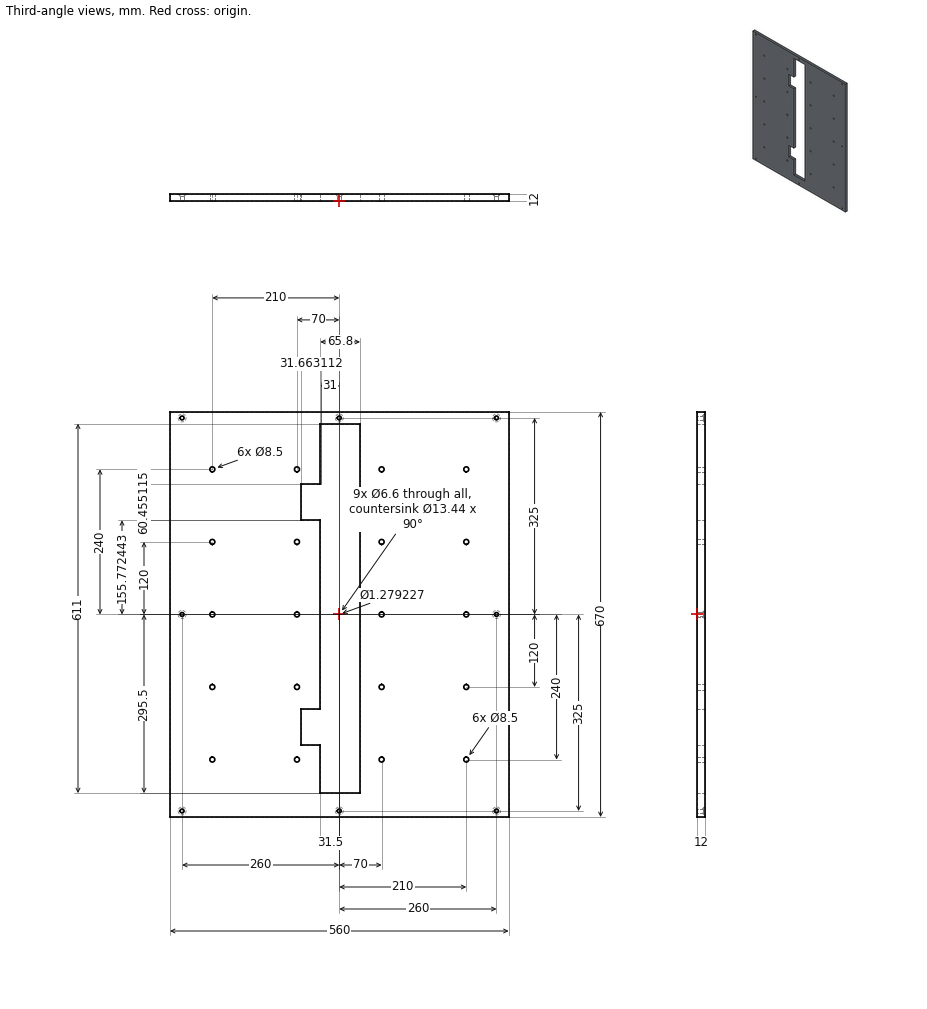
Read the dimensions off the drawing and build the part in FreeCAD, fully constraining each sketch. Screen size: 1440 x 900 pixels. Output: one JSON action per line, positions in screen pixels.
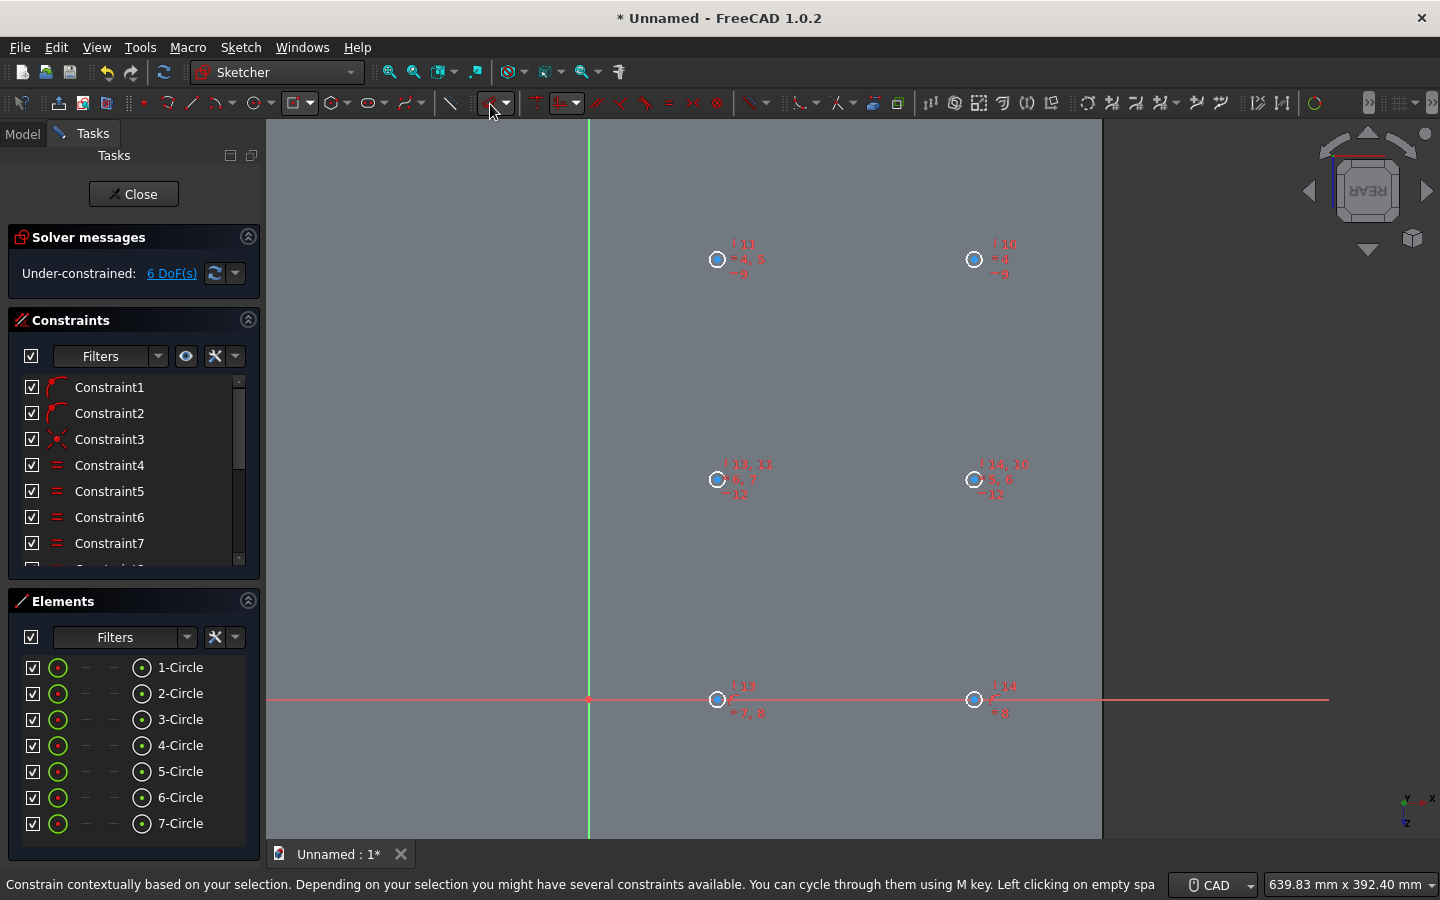
{"action": "scroll", "coordinate": [974, 267], "scroll_direction": "up", "scroll_amount": 5}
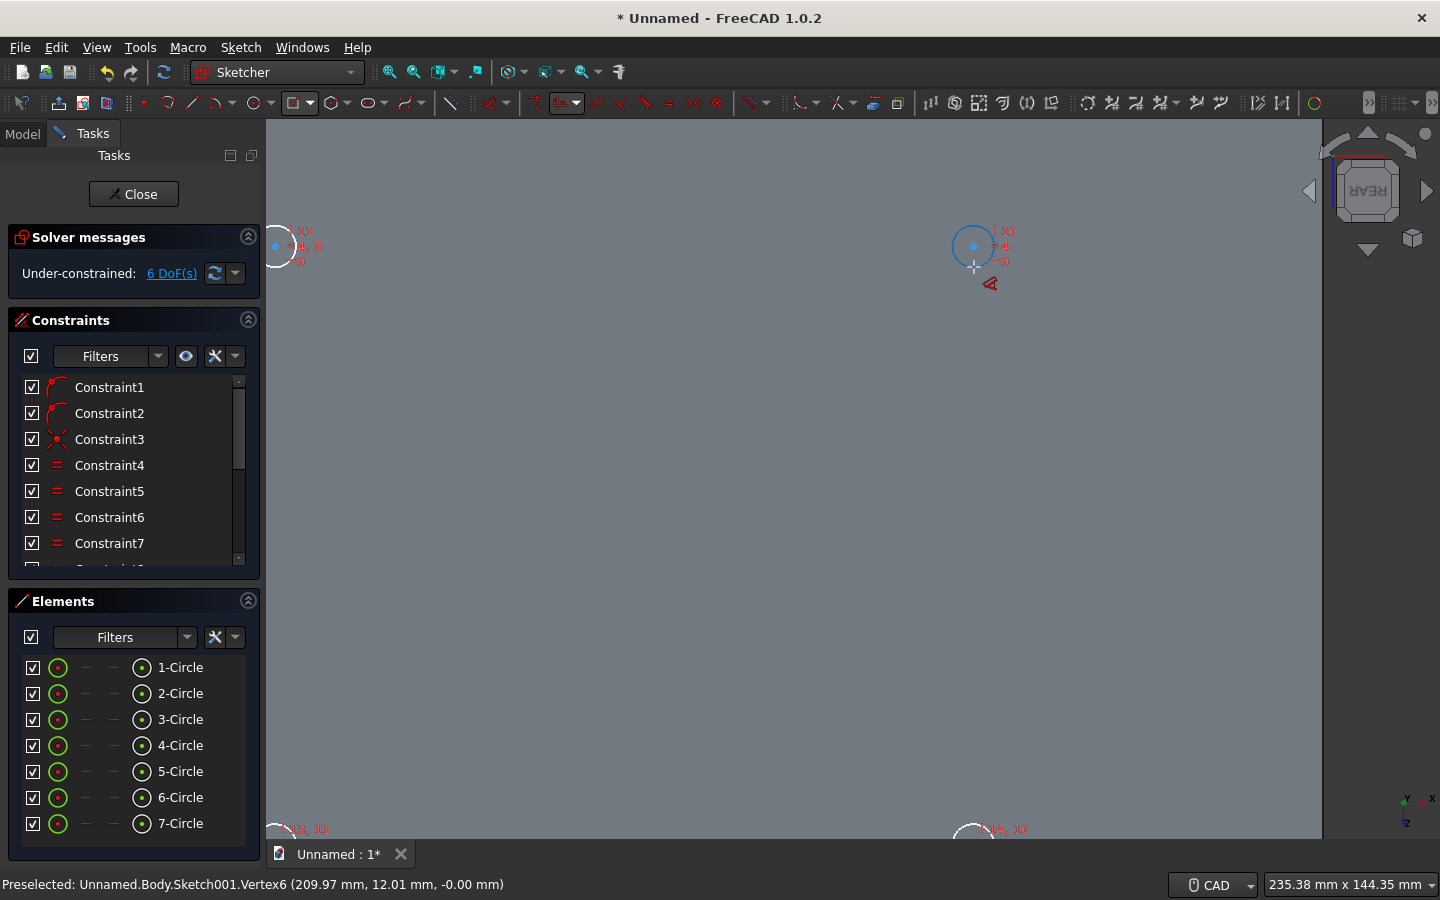
{"action": "left_click", "coordinate": [973, 267]}
{"action": "left_click", "coordinate": [973, 299]}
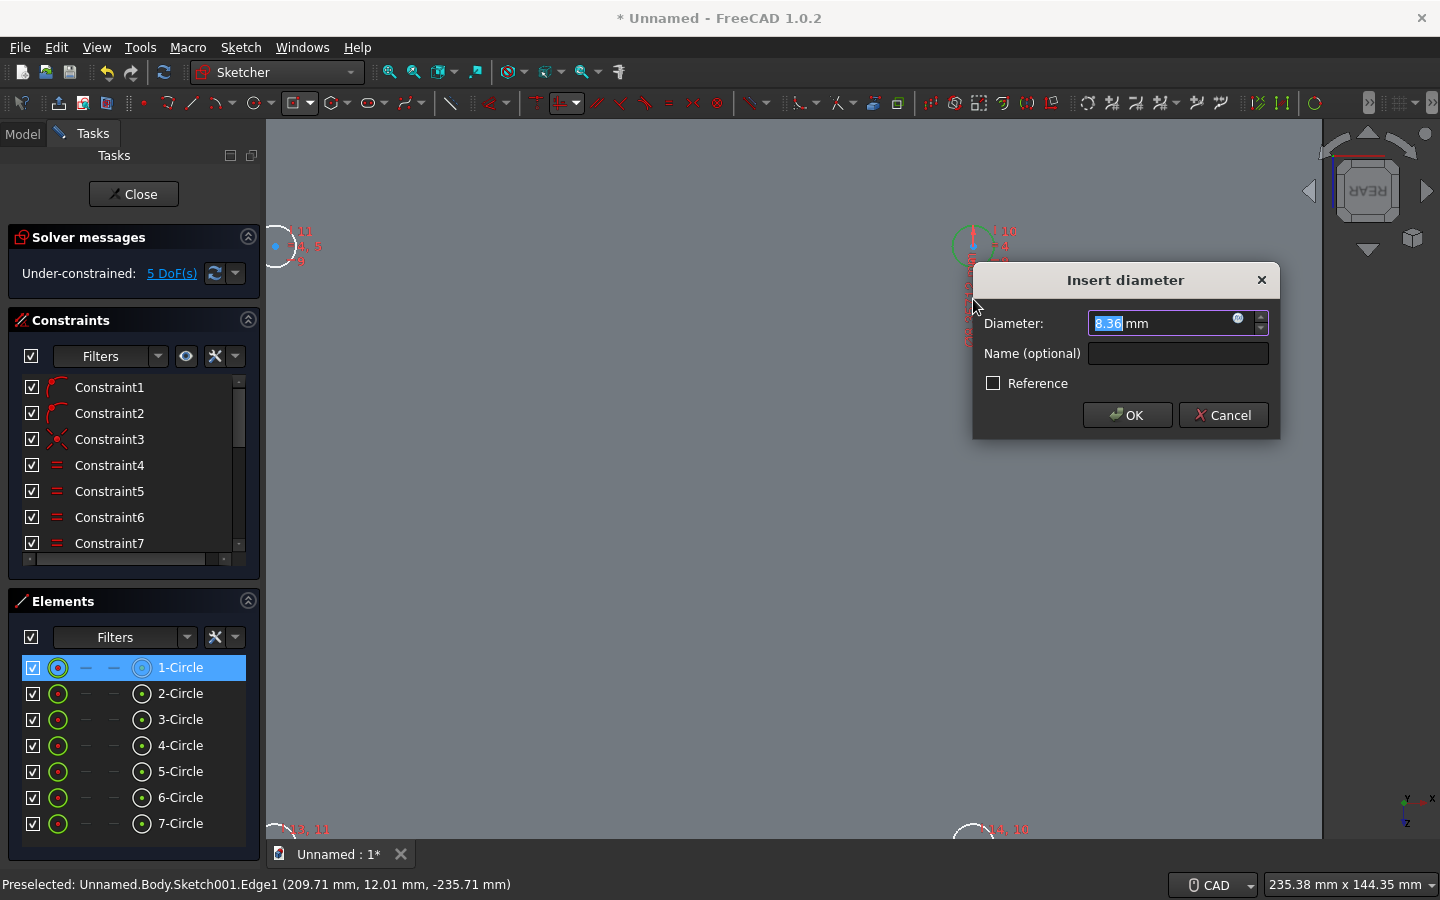
{"action": "type", "text": "8.5"}
{"action": "key", "text": "Return"}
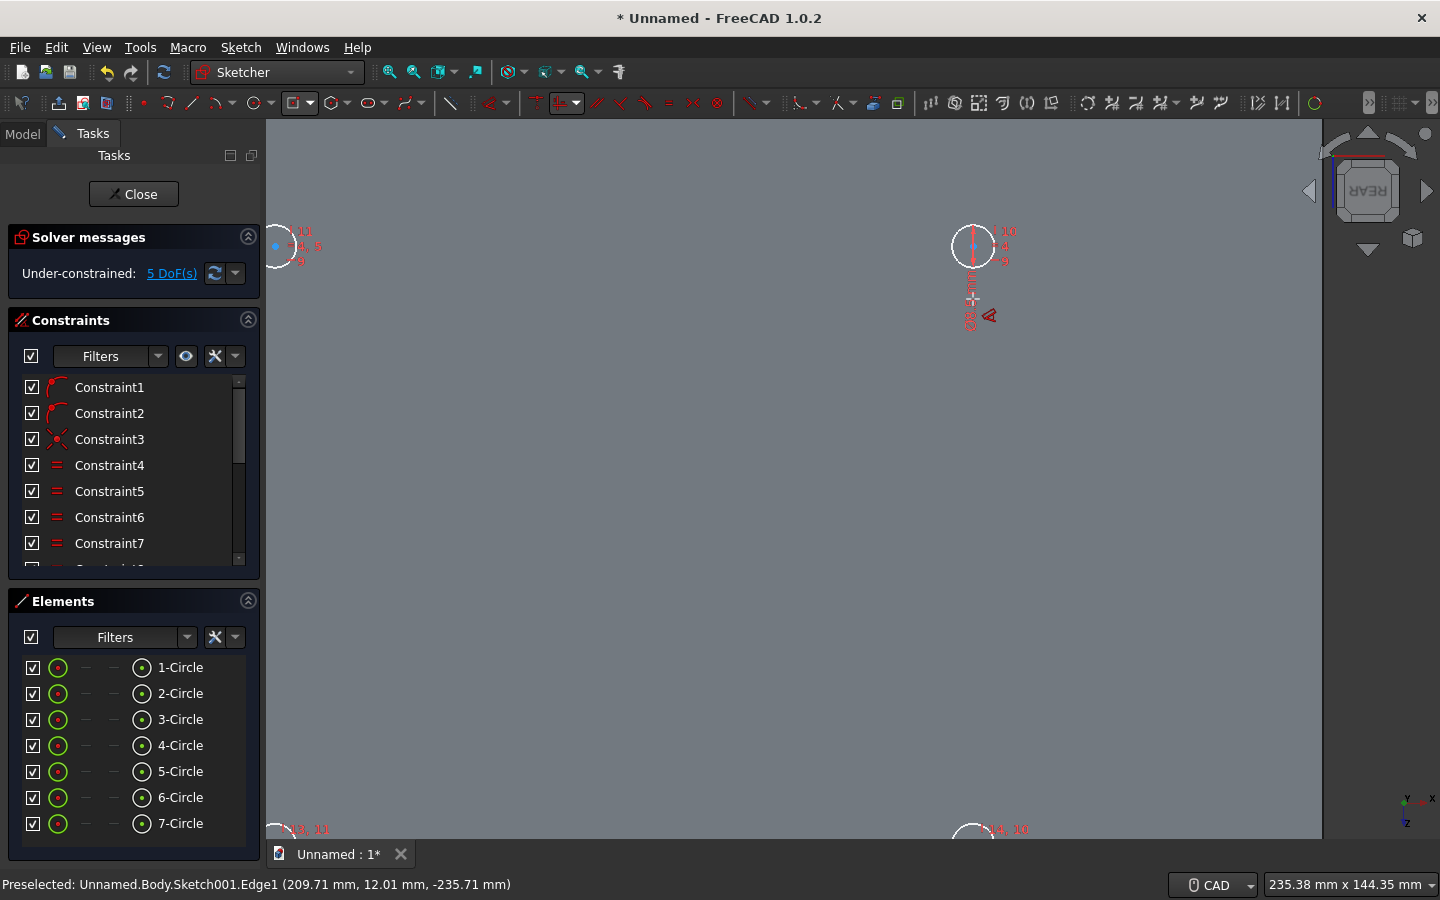
{"action": "scroll", "coordinate": [974, 266], "scroll_direction": "down", "scroll_amount": 5}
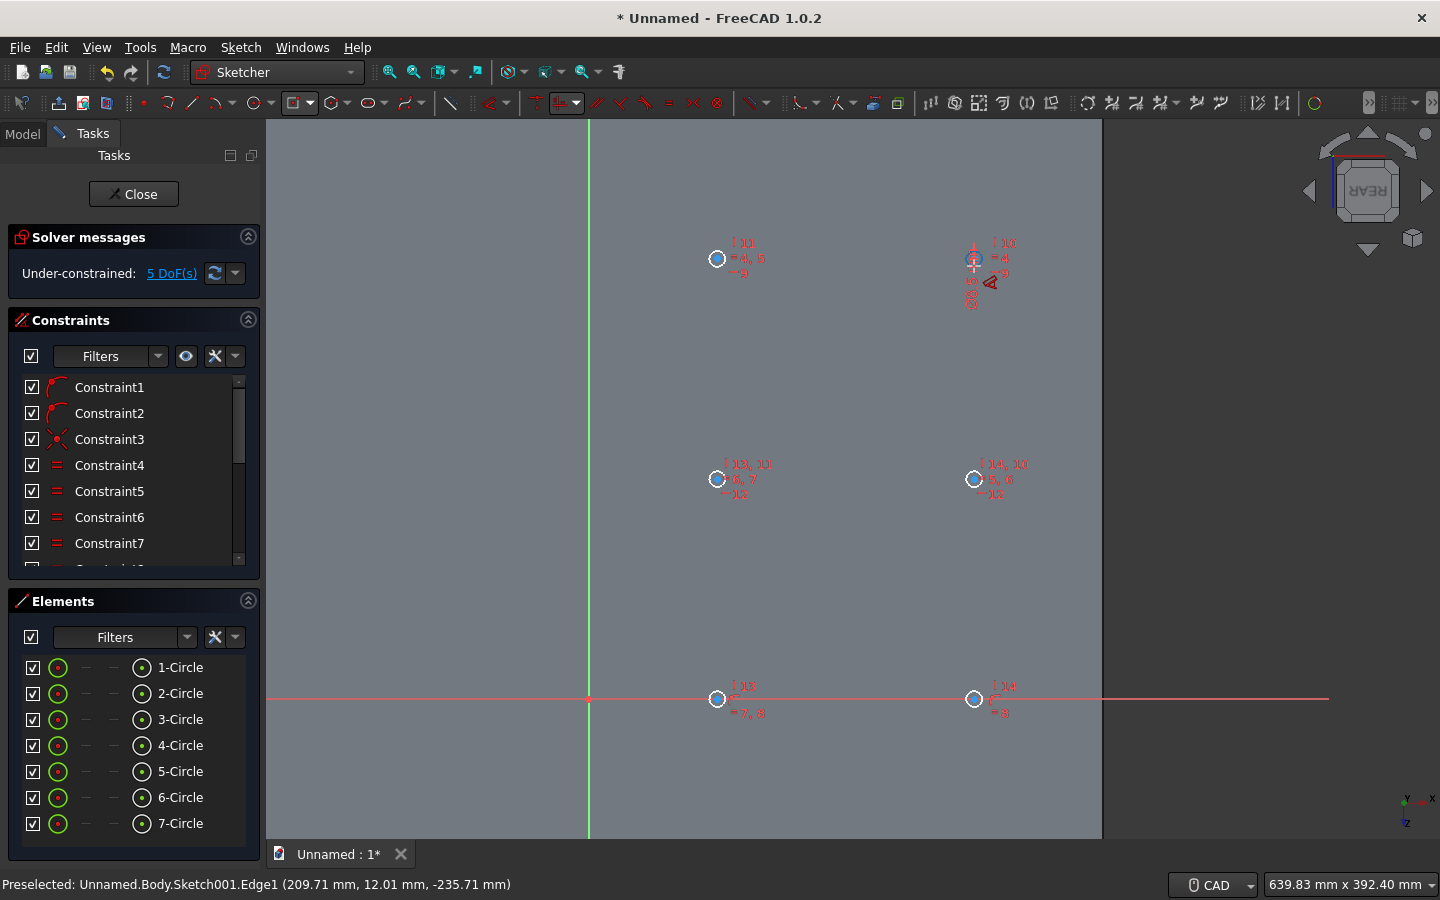
{"action": "scroll", "coordinate": [590, 698], "scroll_direction": "up", "scroll_amount": 15}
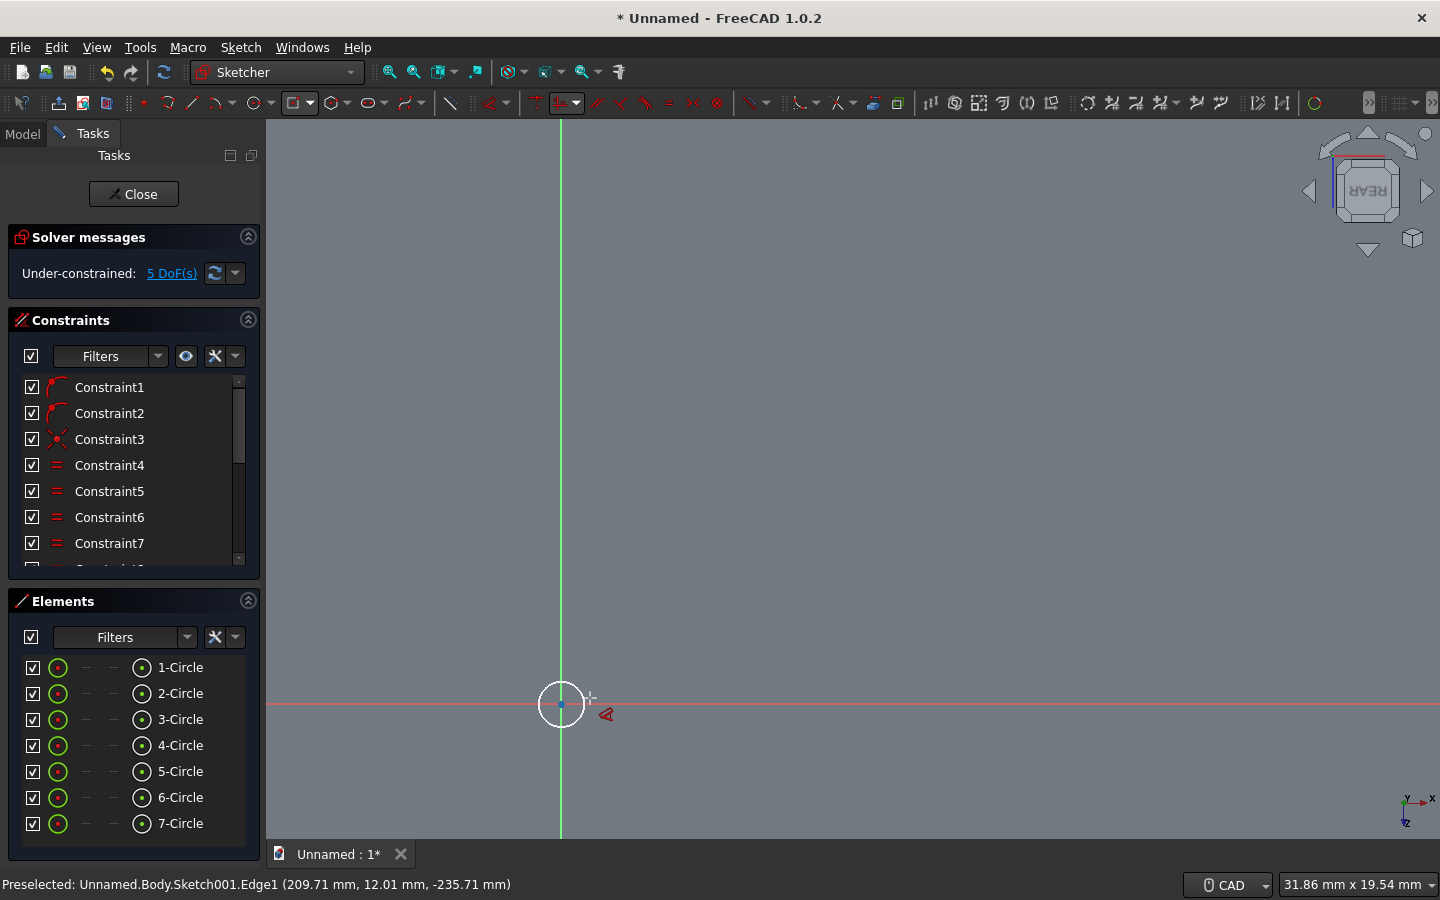
{"action": "left_click", "coordinate": [577, 688]}
{"action": "left_click", "coordinate": [599, 665]}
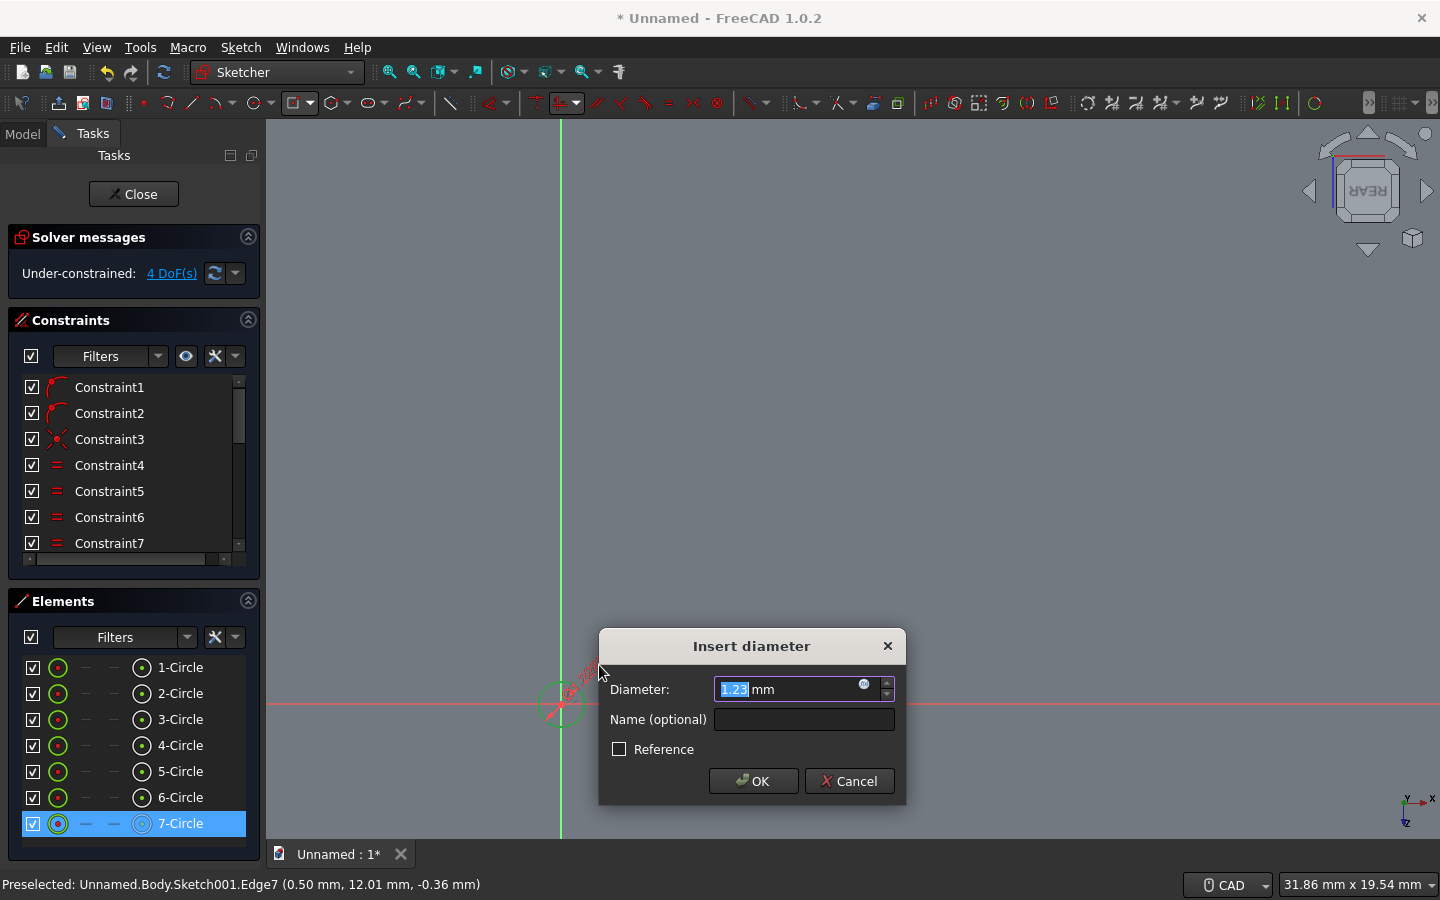
{"action": "type", "text": "1.279227"}
{"action": "key", "text": "Return"}